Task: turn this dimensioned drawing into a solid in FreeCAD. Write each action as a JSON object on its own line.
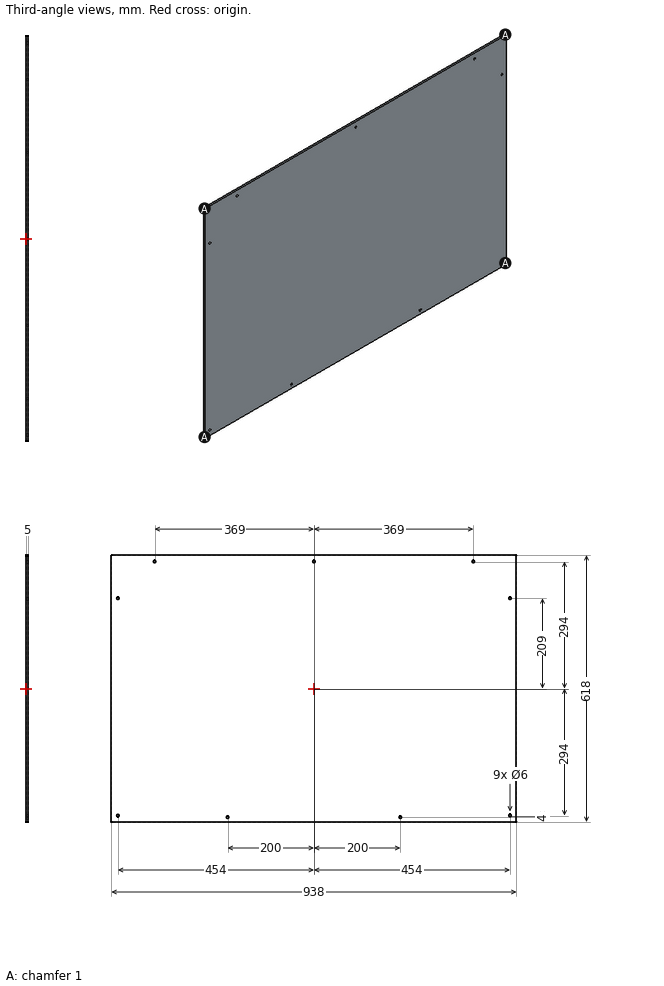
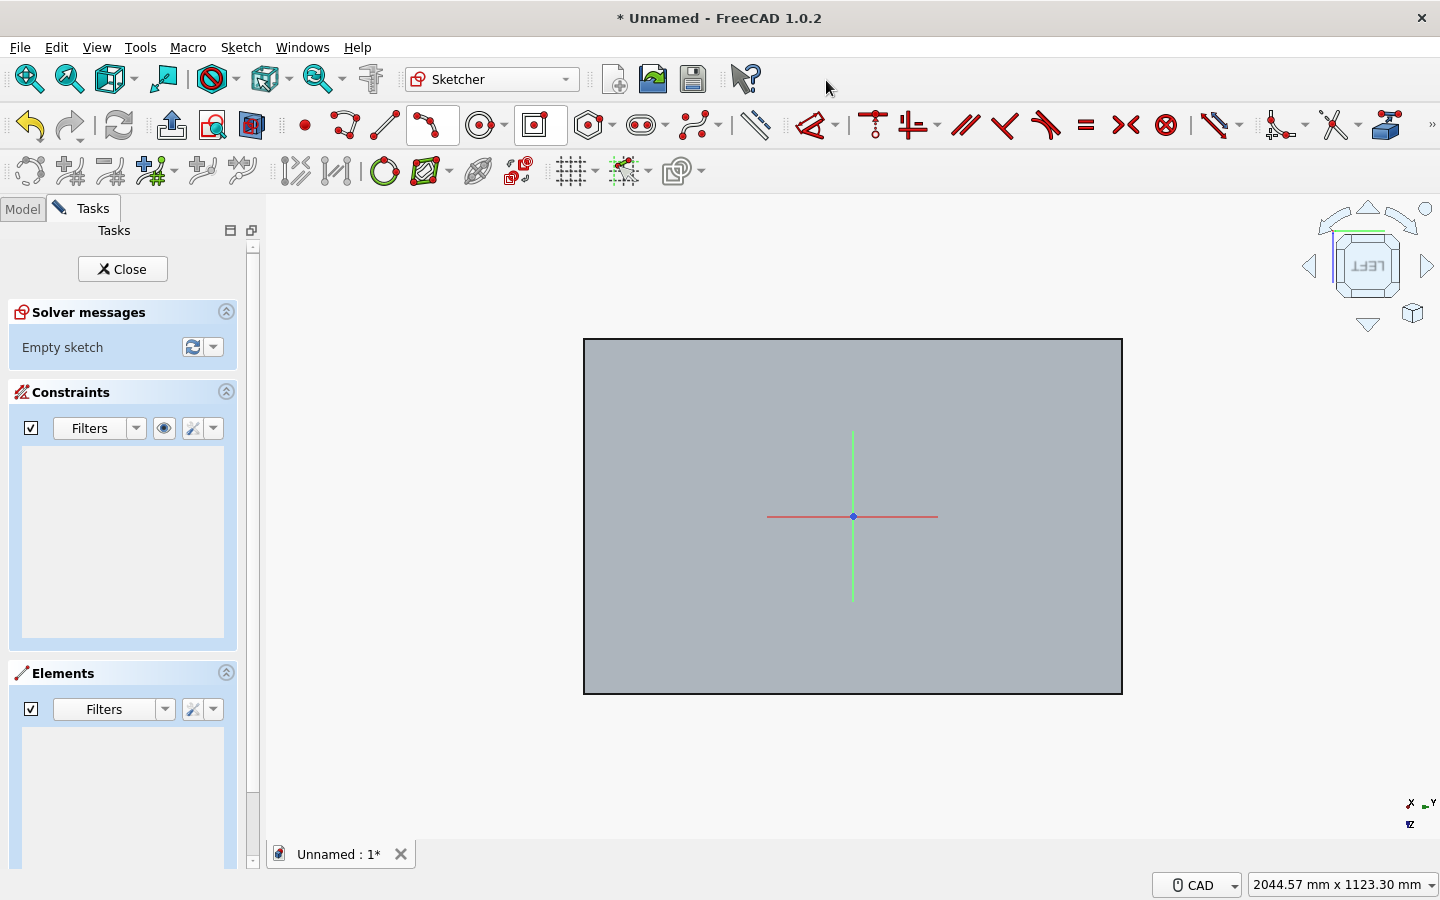
{"action": "left_click", "coordinate": [480, 126]}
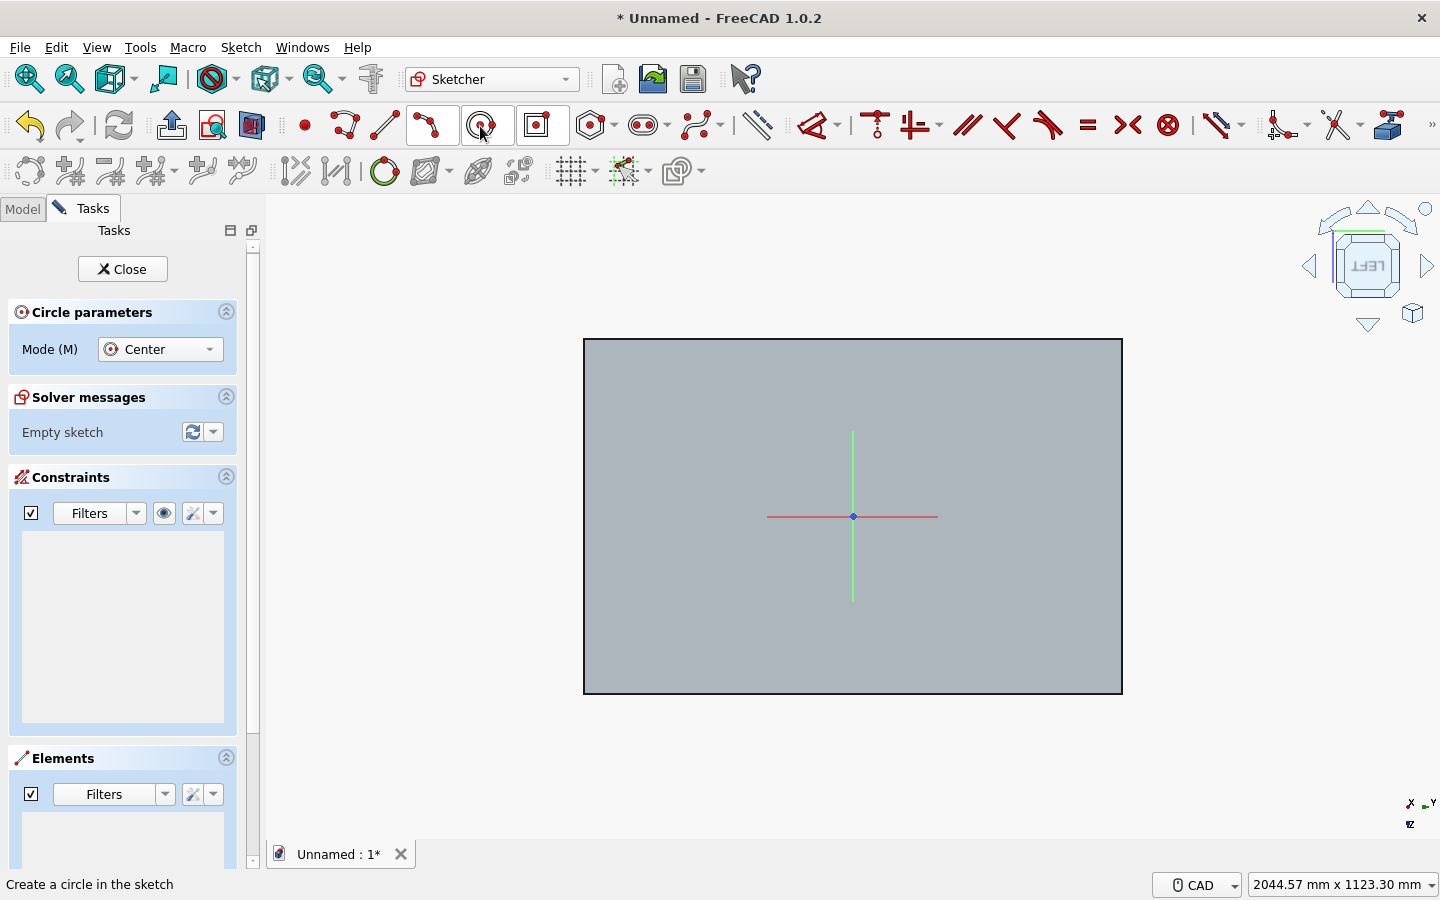
{"action": "scroll", "coordinate": [1114, 348], "scroll_direction": "up", "scroll_amount": 13}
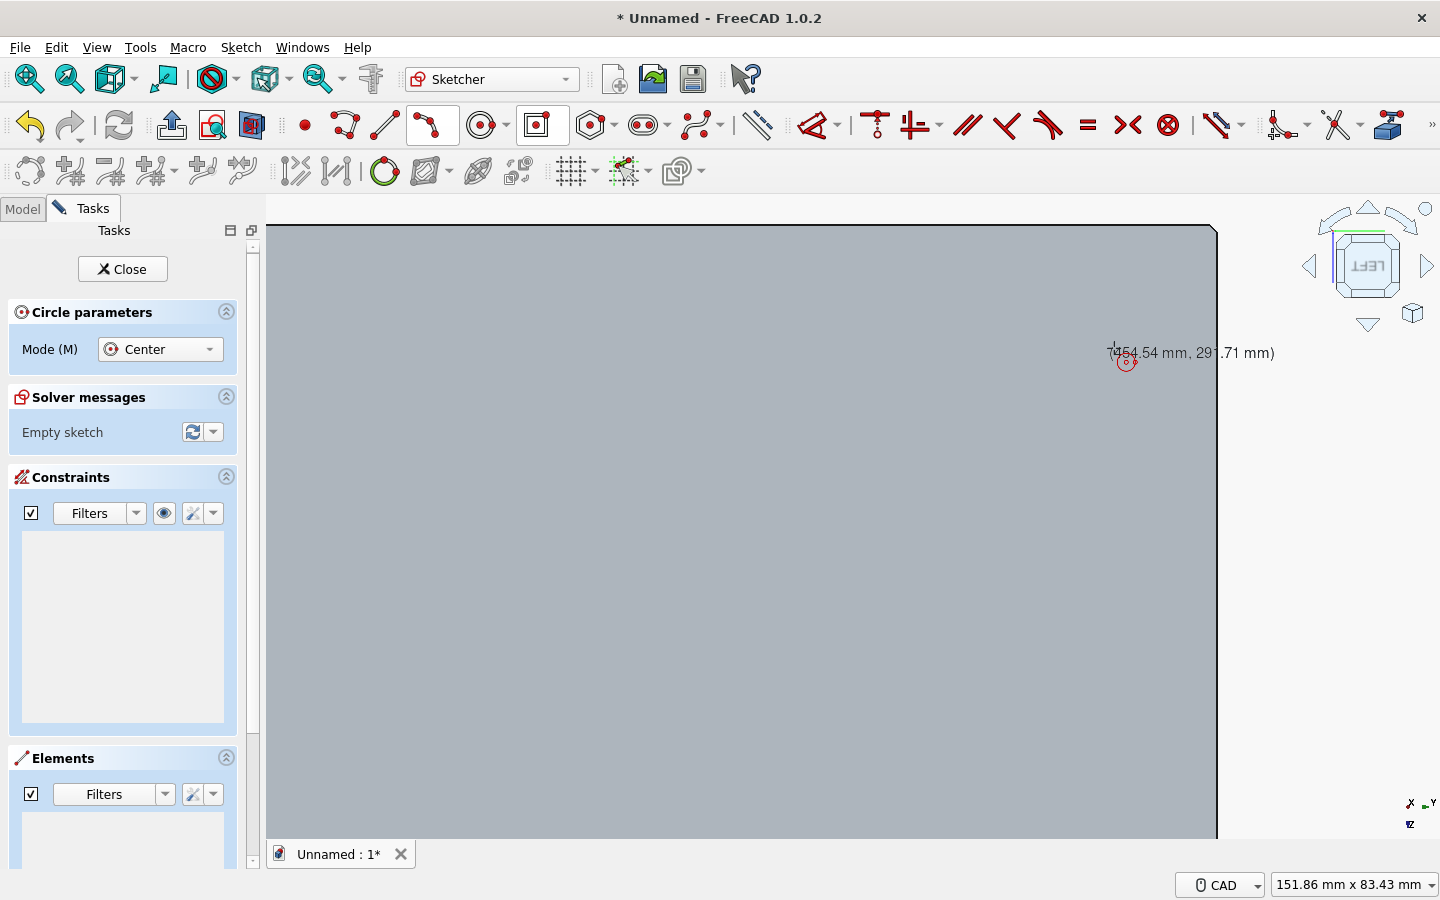
{"action": "scroll", "coordinate": [1103, 309], "scroll_direction": "down", "scroll_amount": 12}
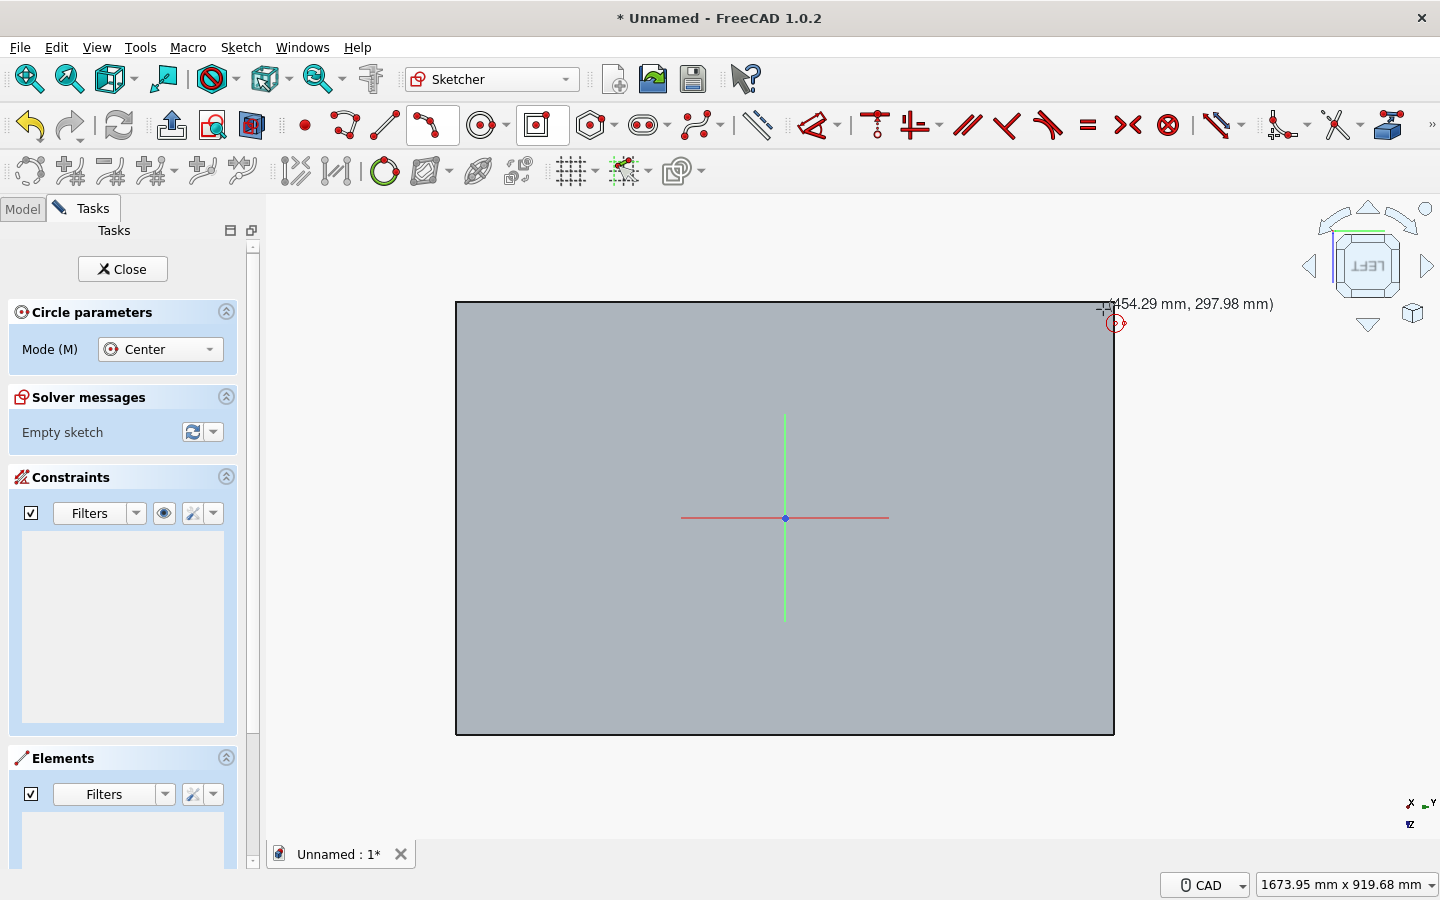
{"action": "left_click", "coordinate": [1103, 312]}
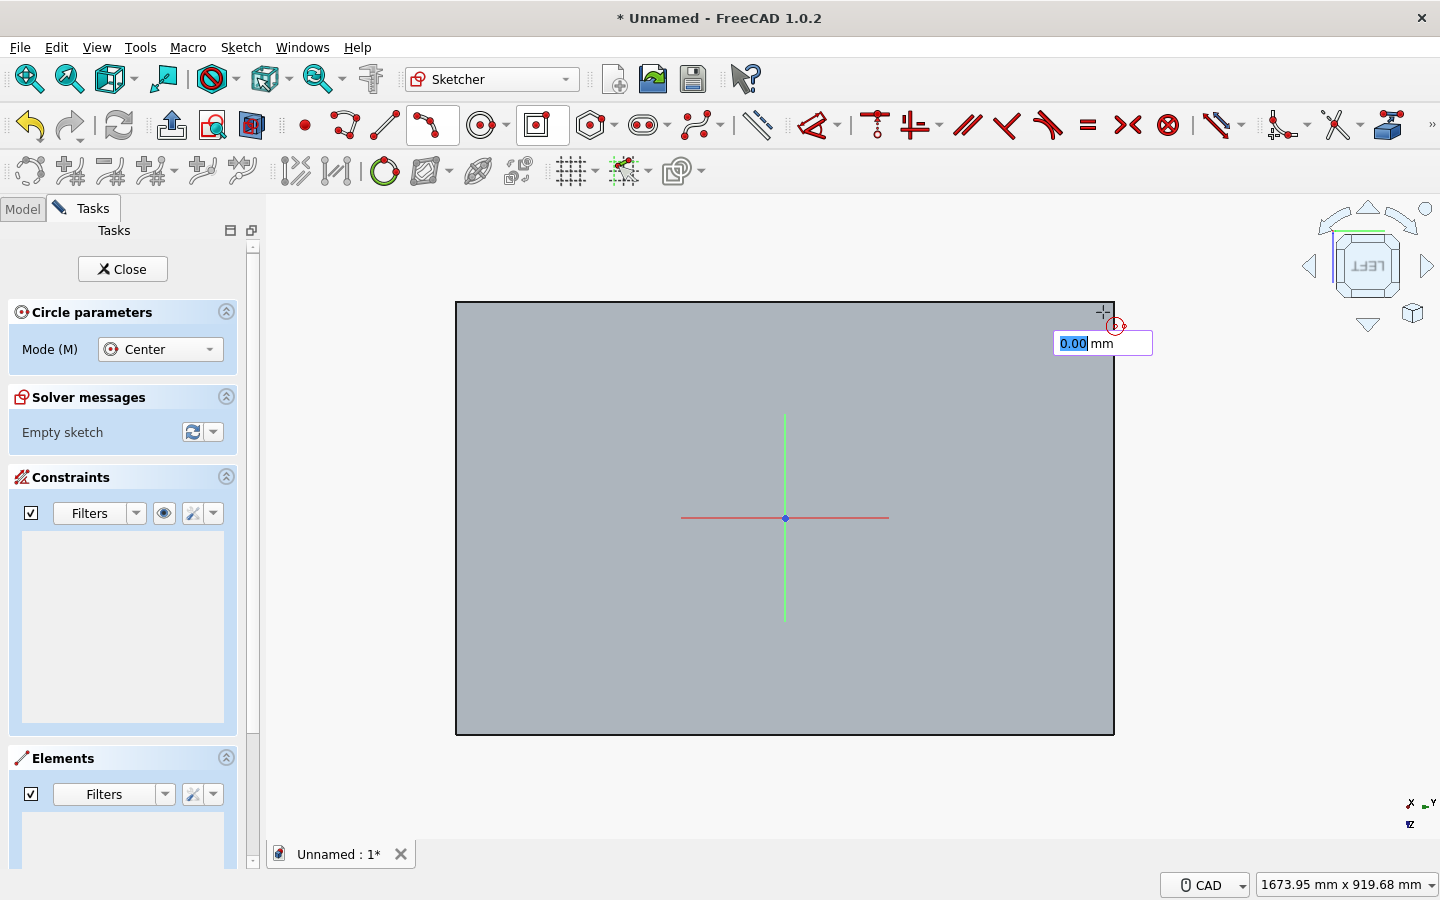
{"action": "scroll", "coordinate": [1105, 311], "scroll_direction": "up", "scroll_amount": 11}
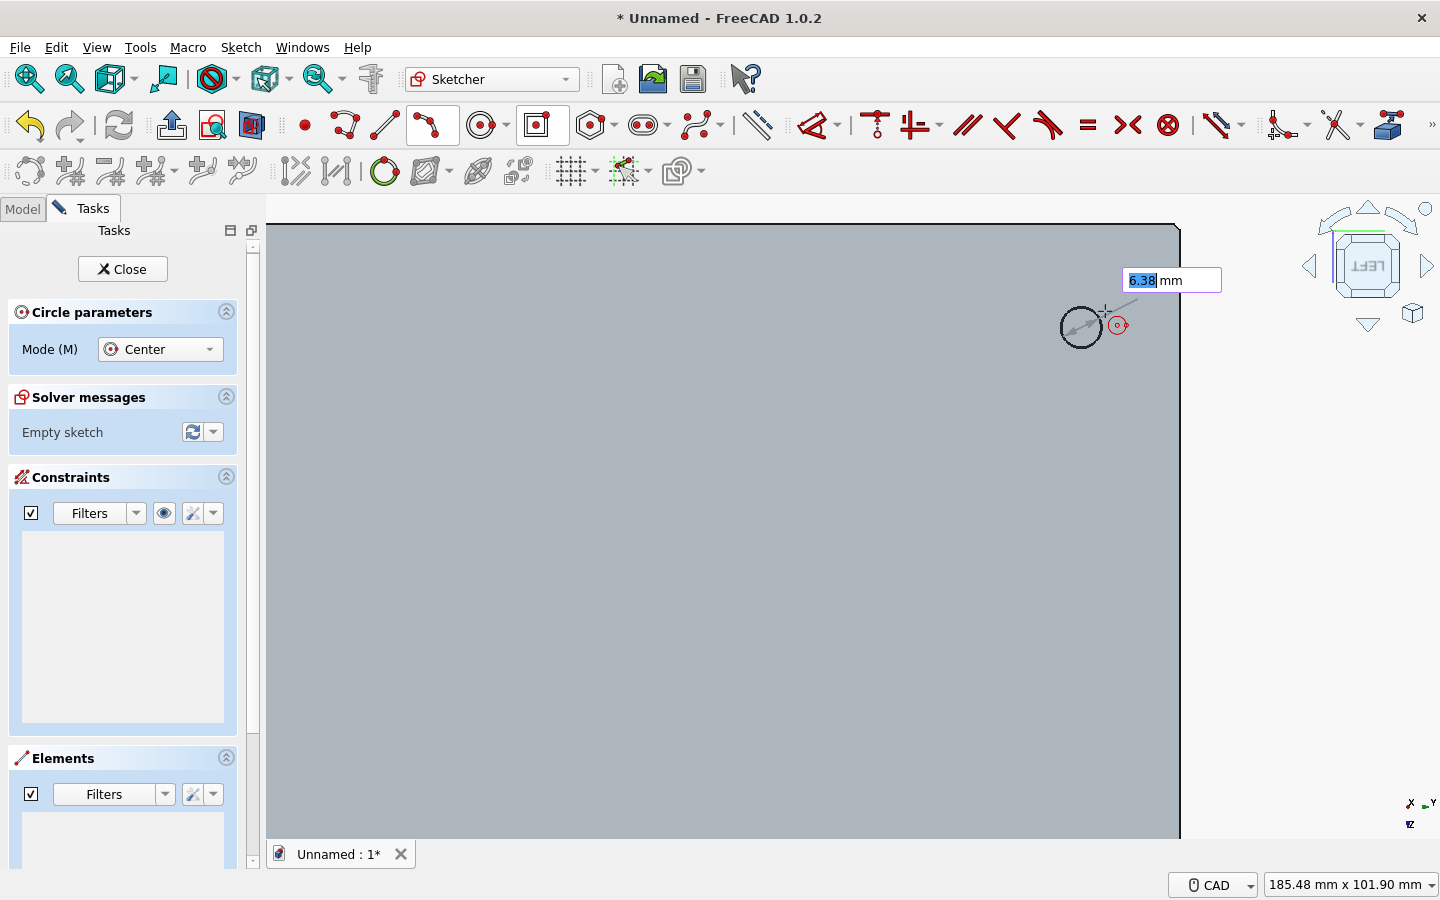
{"action": "left_click", "coordinate": [1099, 306]}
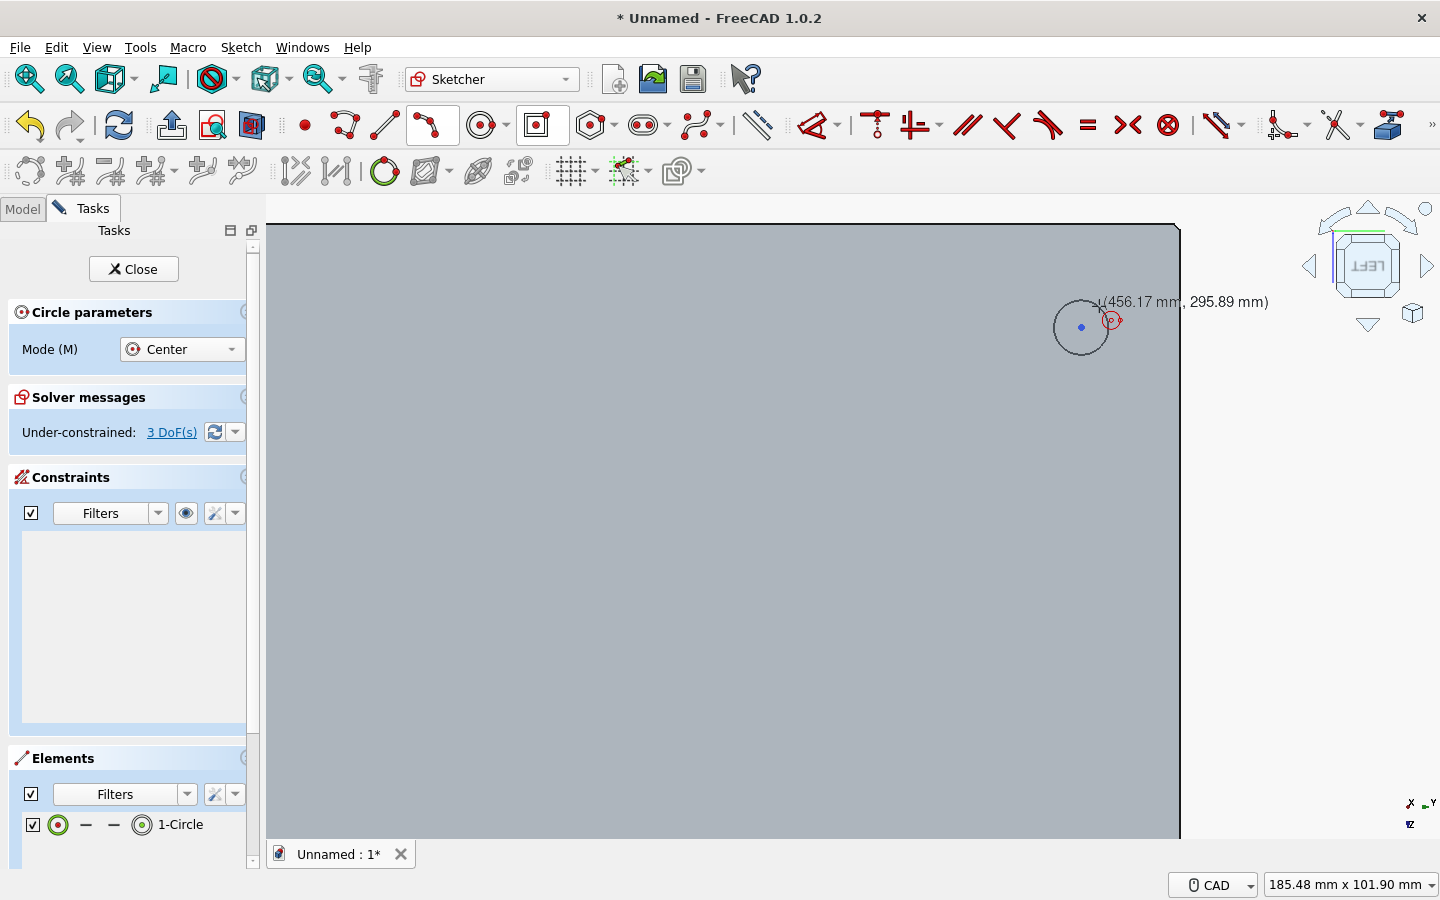
{"action": "scroll", "coordinate": [1105, 311], "scroll_direction": "down", "scroll_amount": 11}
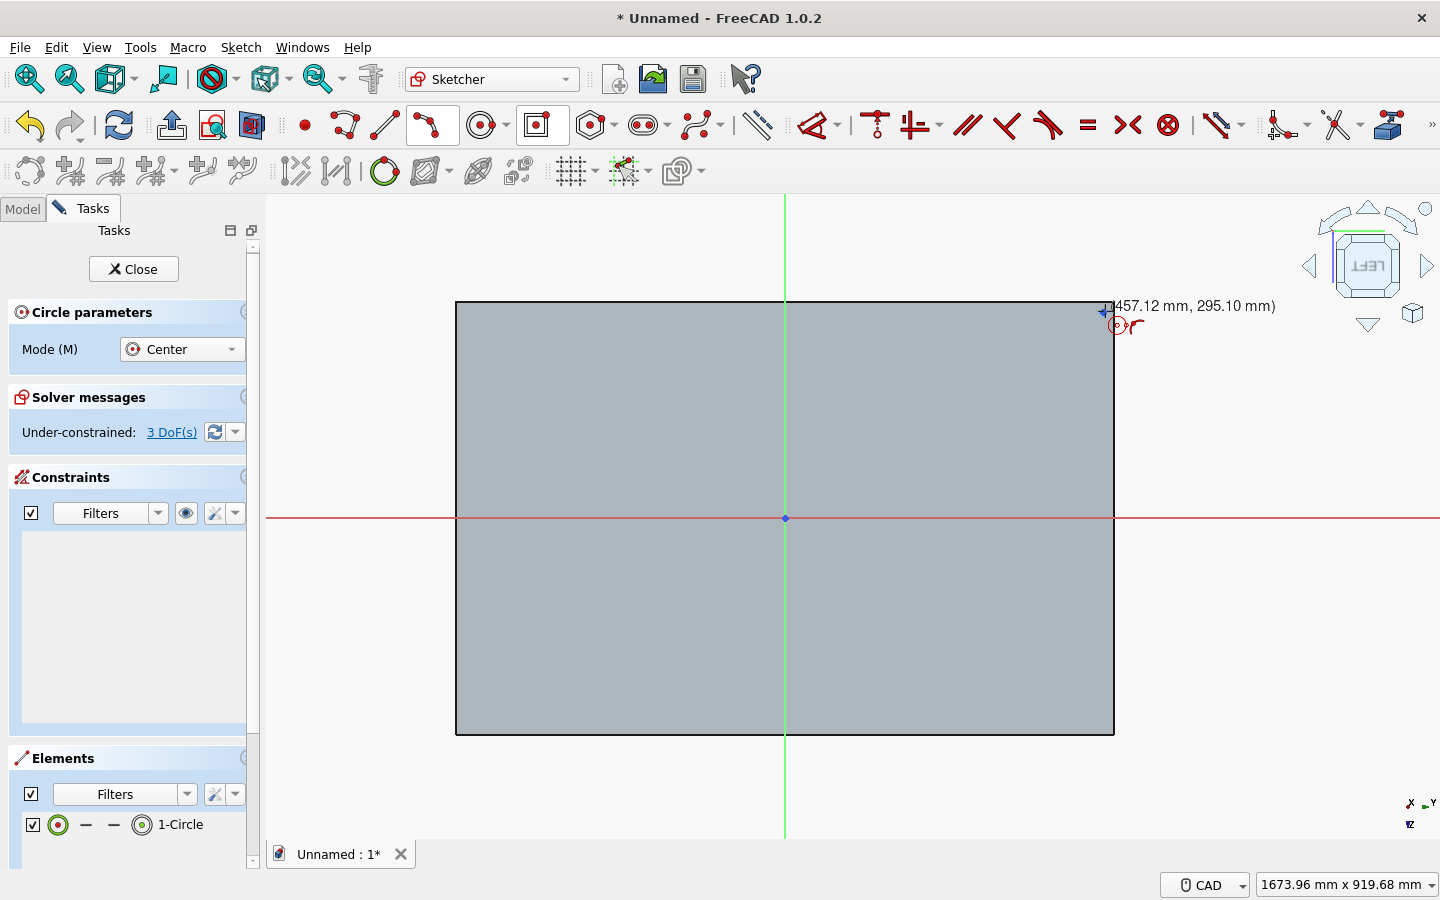
{"action": "scroll", "coordinate": [467, 312], "scroll_direction": "up", "scroll_amount": 12}